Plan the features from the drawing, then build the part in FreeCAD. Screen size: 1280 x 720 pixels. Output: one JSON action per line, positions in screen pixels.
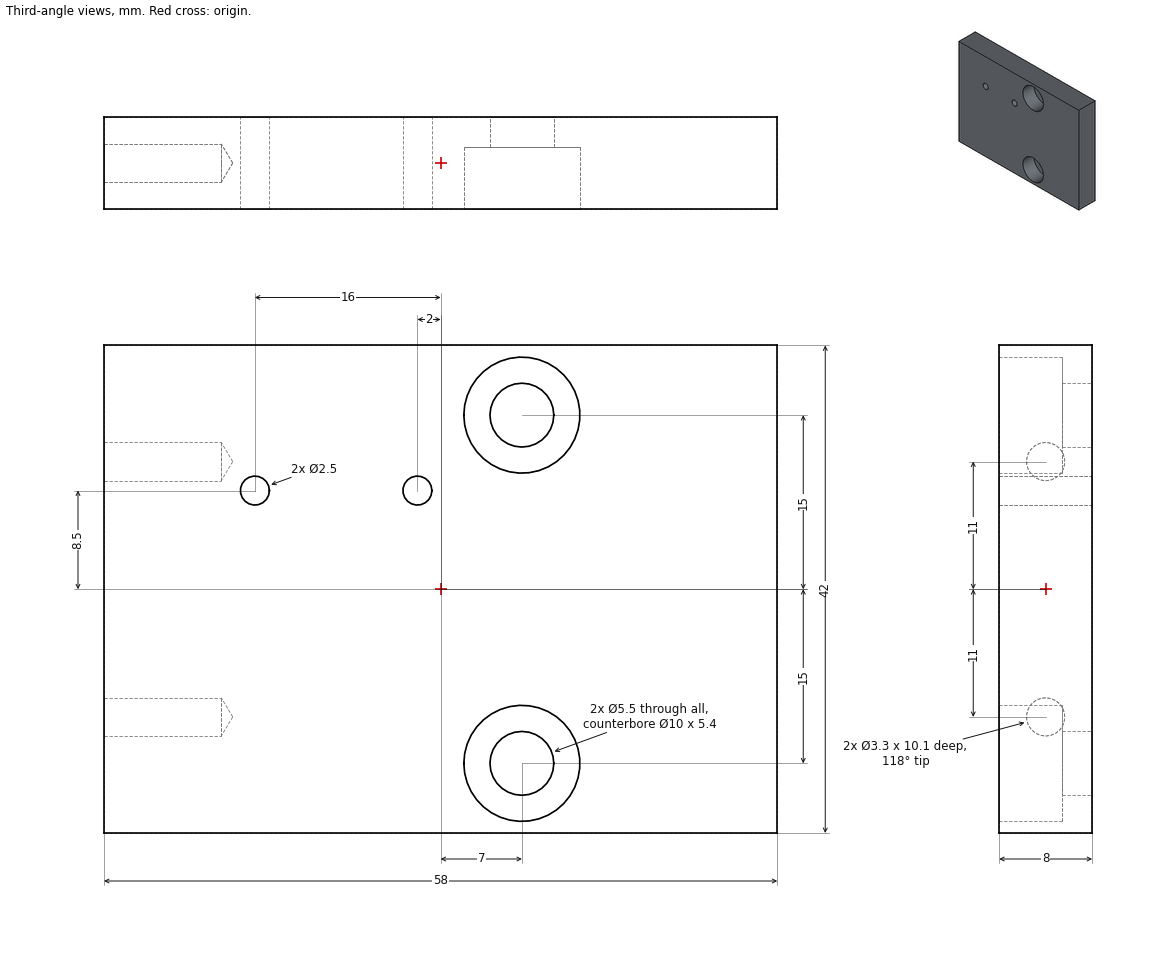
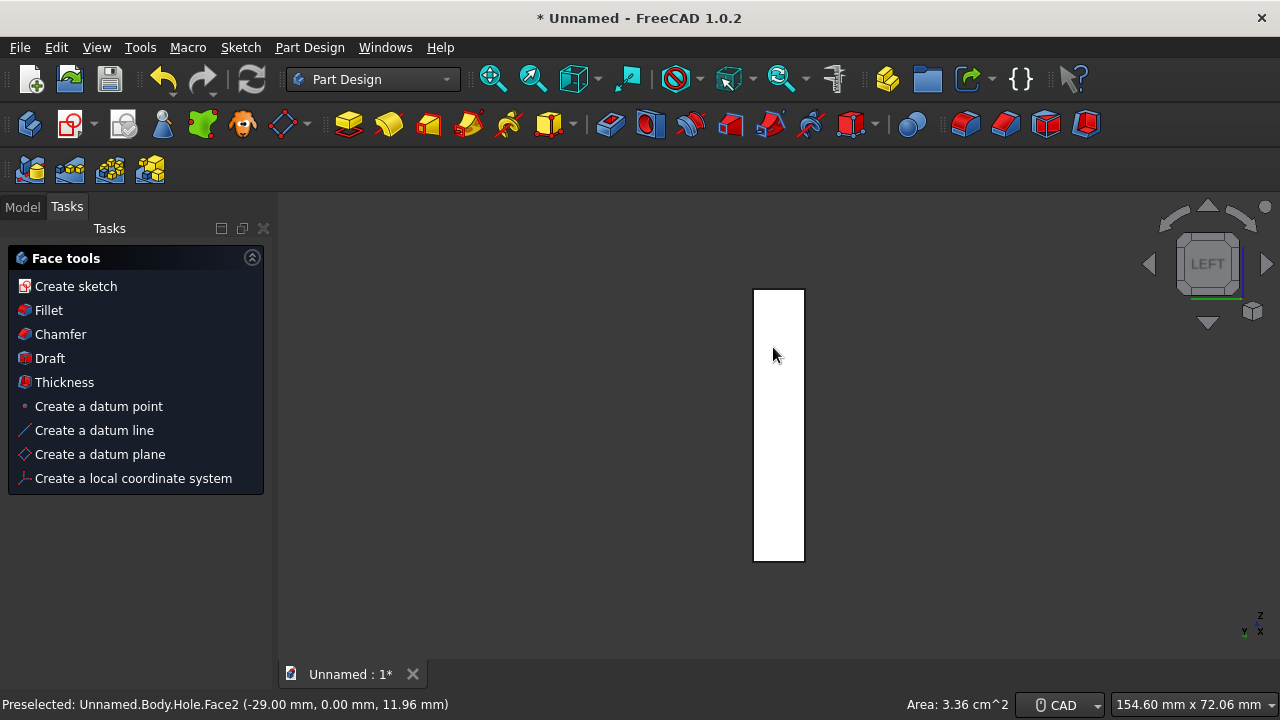
{"action": "left_click", "coordinate": [70, 124]}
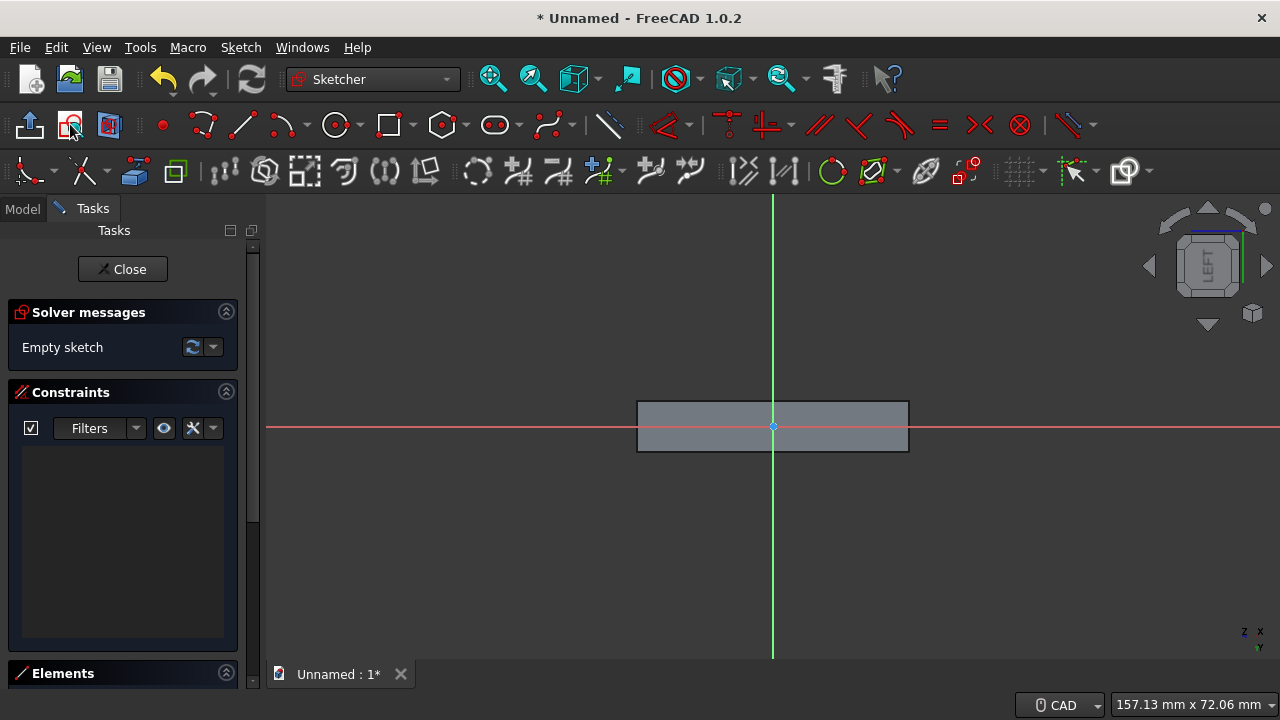
{"action": "scroll", "coordinate": [803, 427], "scroll_direction": "up", "scroll_amount": 6}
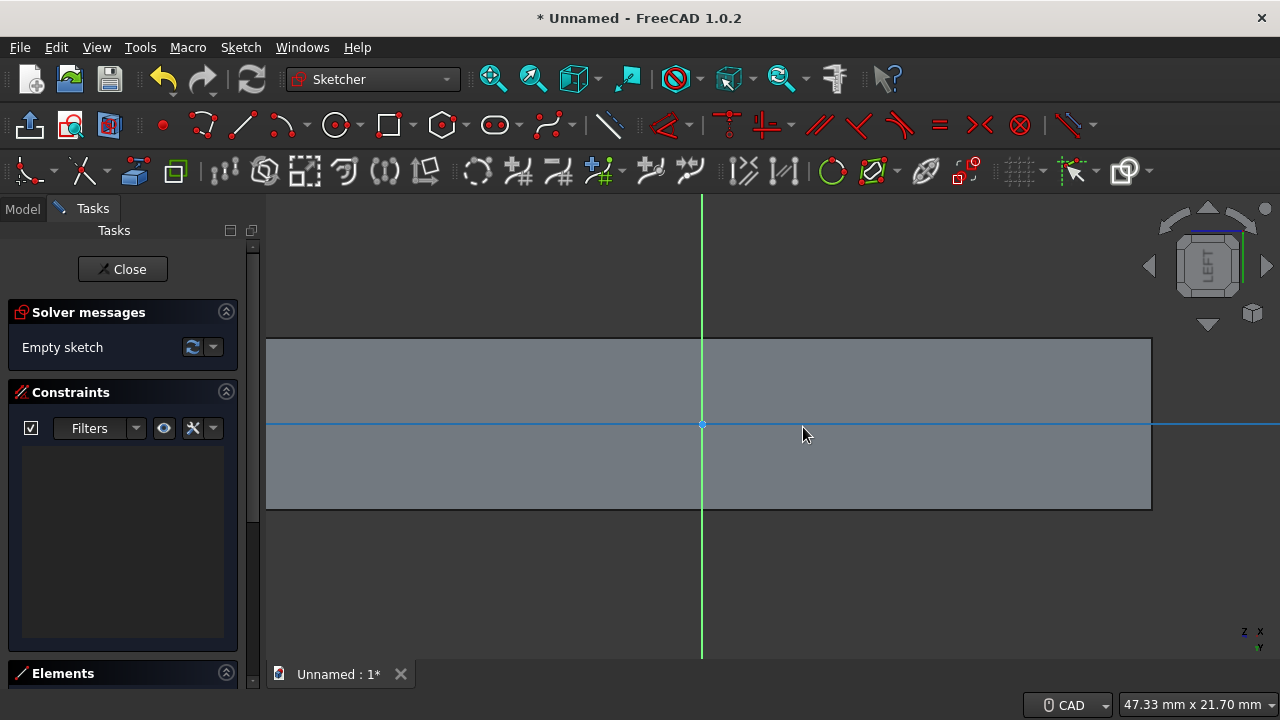
{"action": "left_click", "coordinate": [336, 126]}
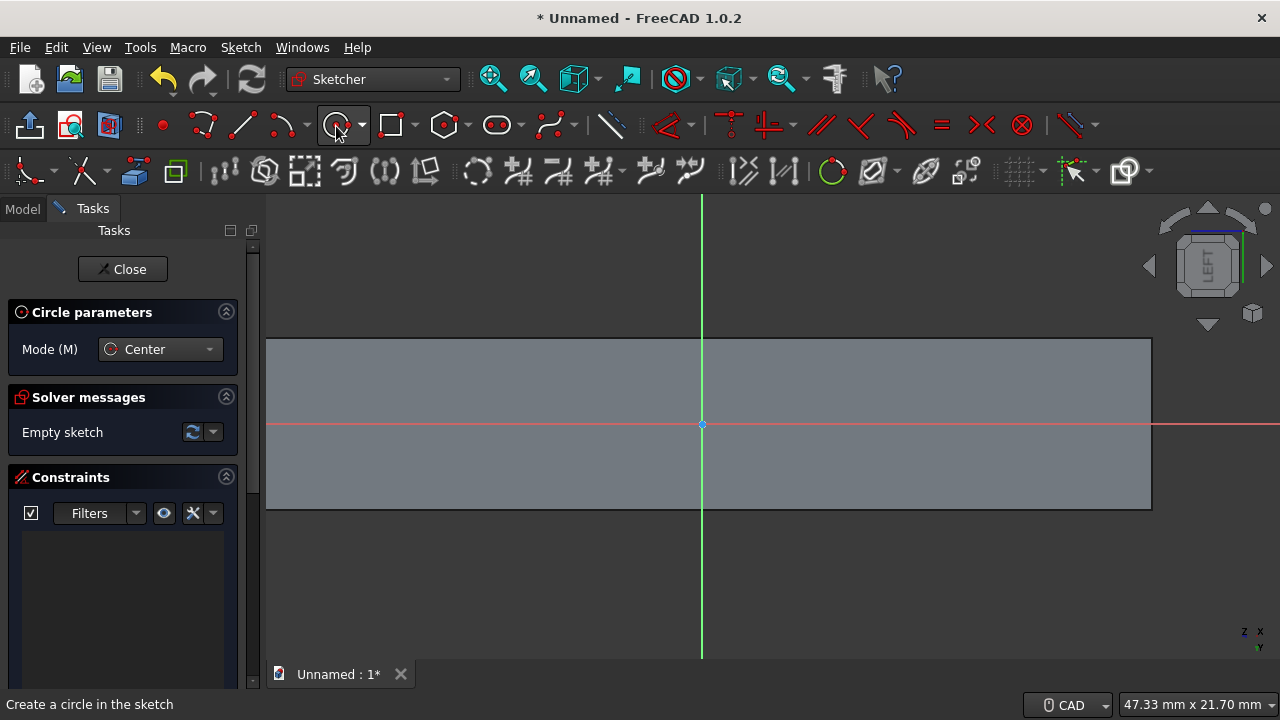
{"action": "left_click", "coordinate": [938, 424]}
{"action": "left_click", "coordinate": [963, 399]}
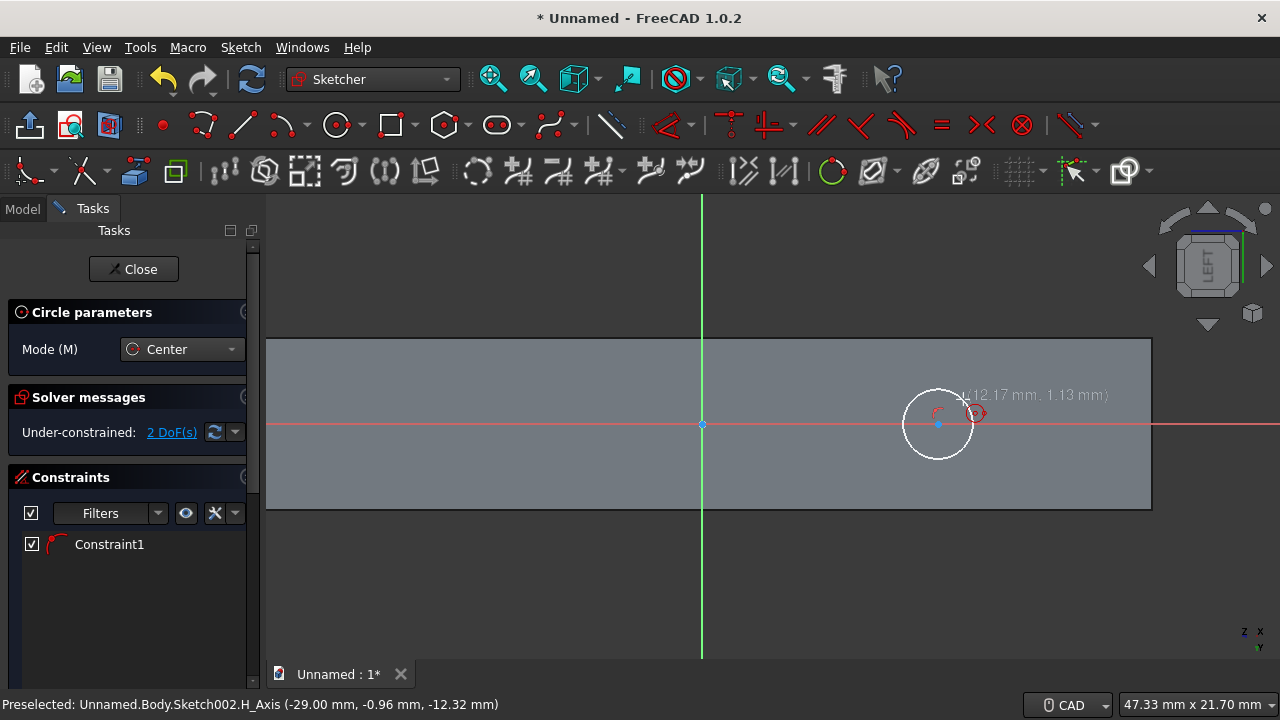
{"action": "left_click", "coordinate": [466, 424]}
{"action": "left_click", "coordinate": [491, 399]}
{"action": "key", "text": "Escape"}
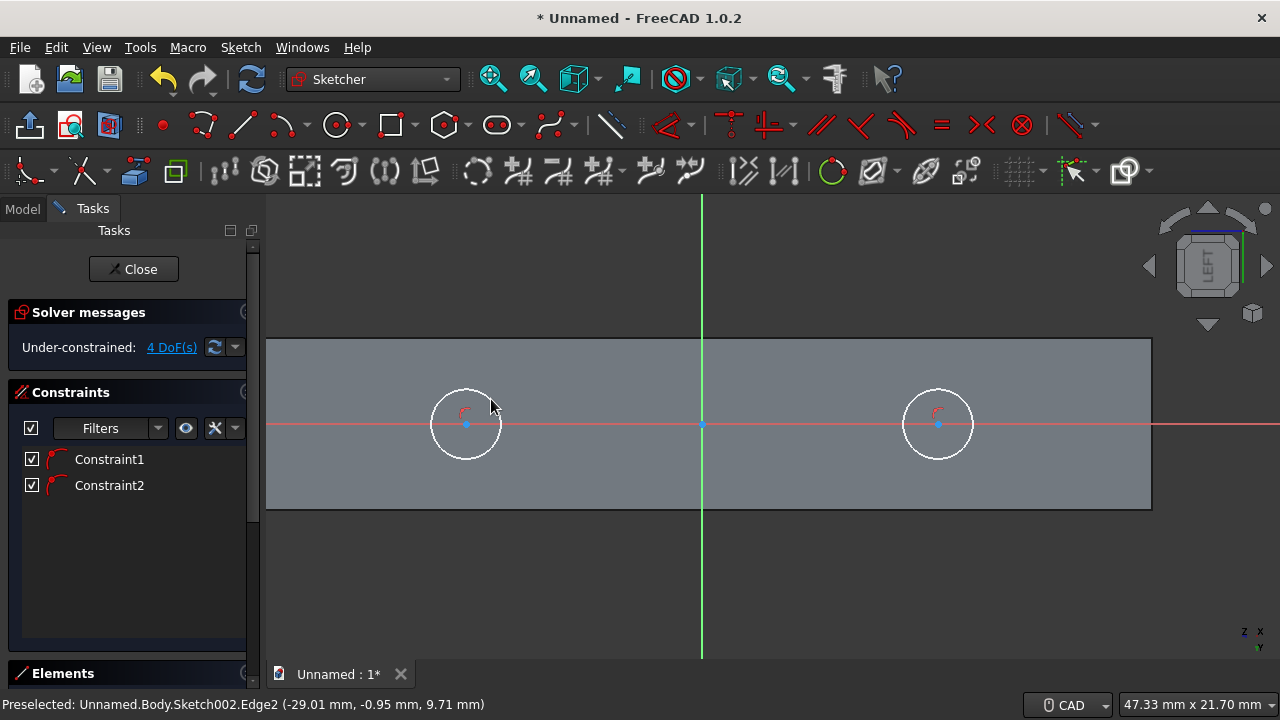
{"action": "left_click", "coordinate": [963, 400]}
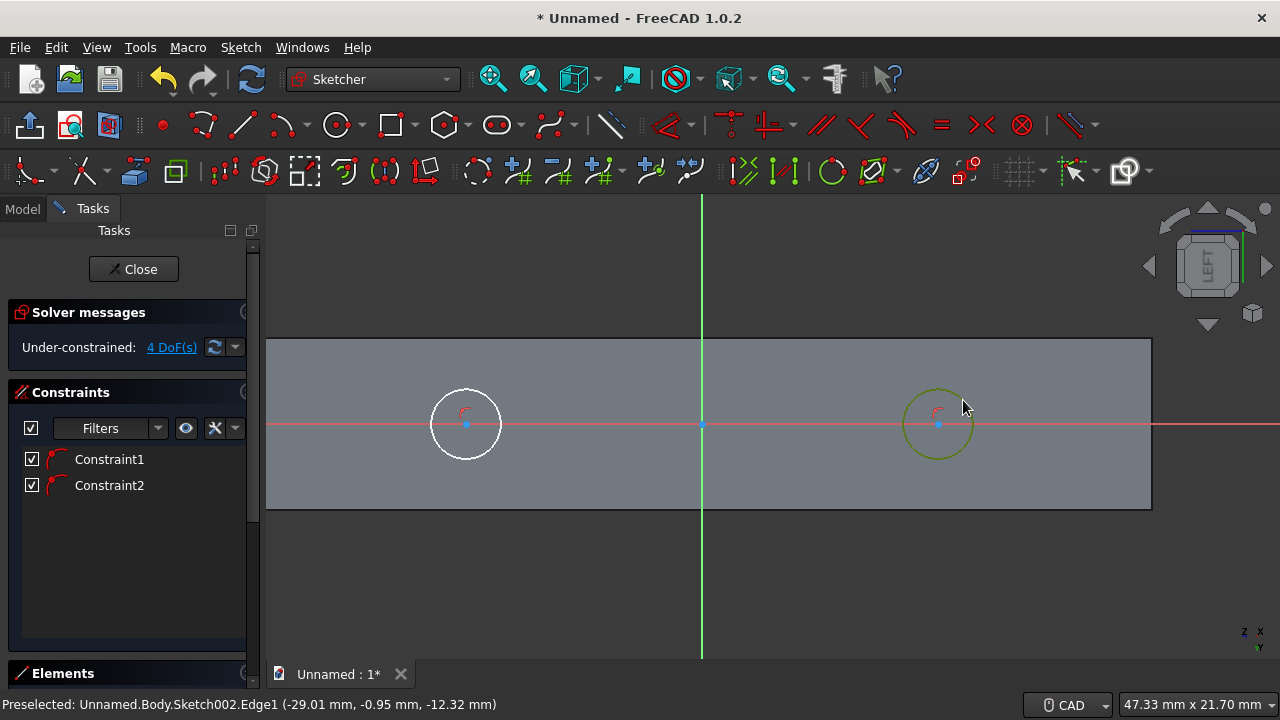
{"action": "left_click", "coordinate": [491, 400]}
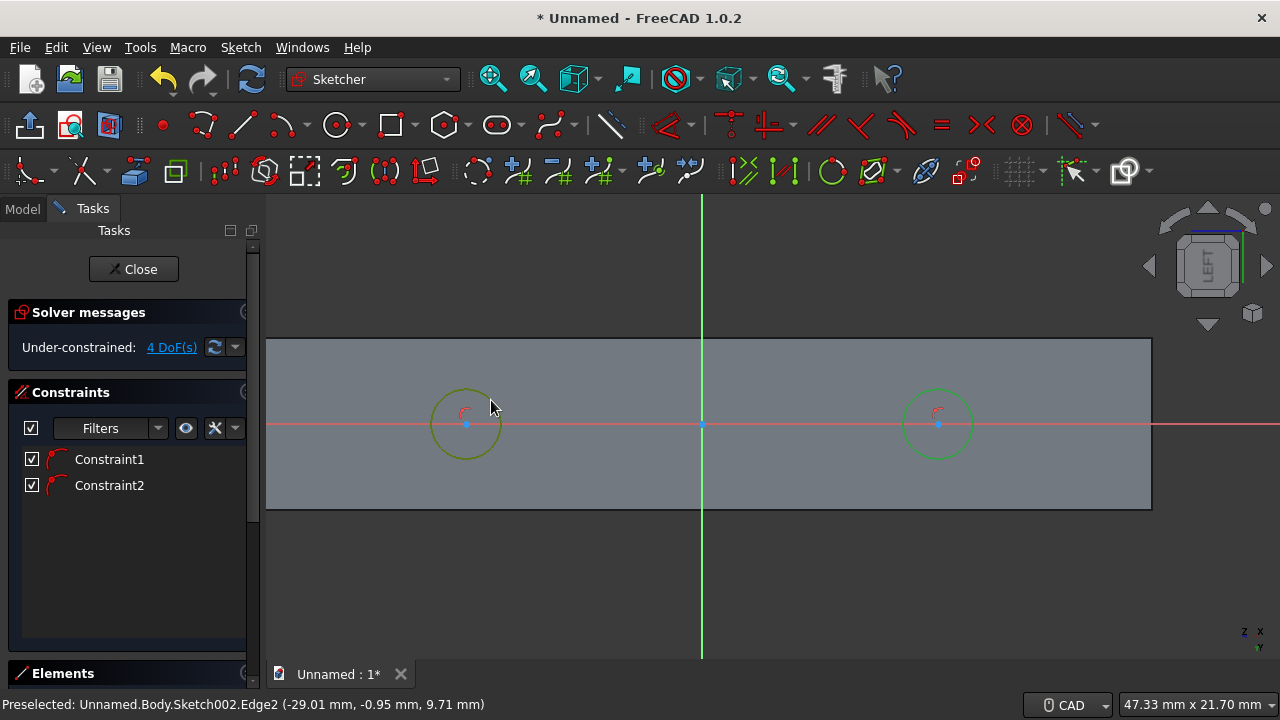
{"action": "left_click", "coordinate": [942, 126]}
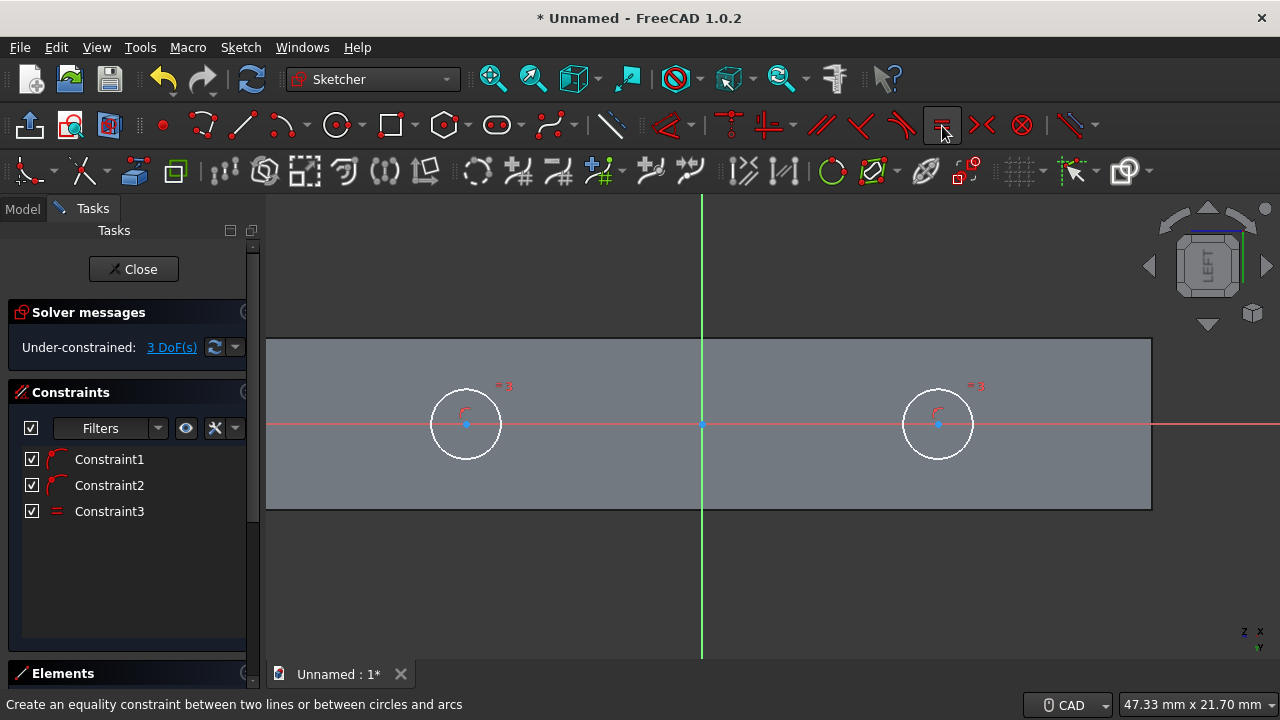
{"action": "left_click", "coordinate": [666, 126]}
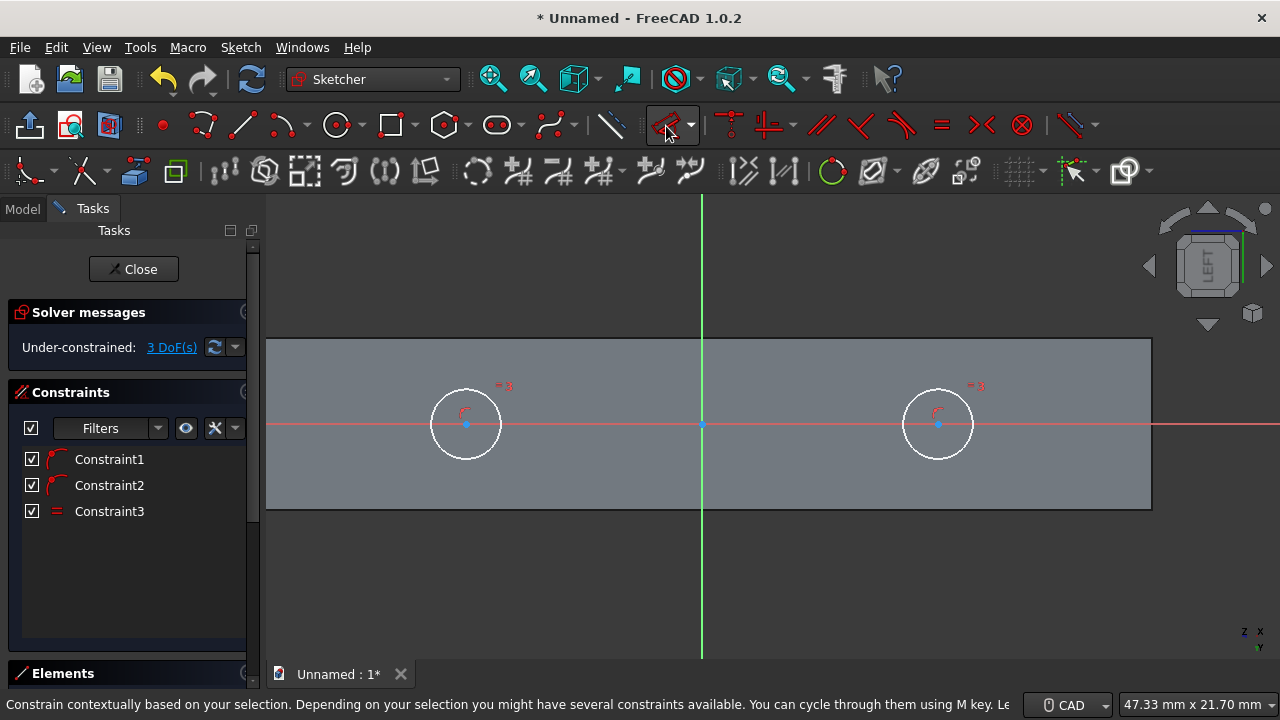
{"action": "left_click", "coordinate": [963, 400]}
{"action": "left_click", "coordinate": [986, 378]}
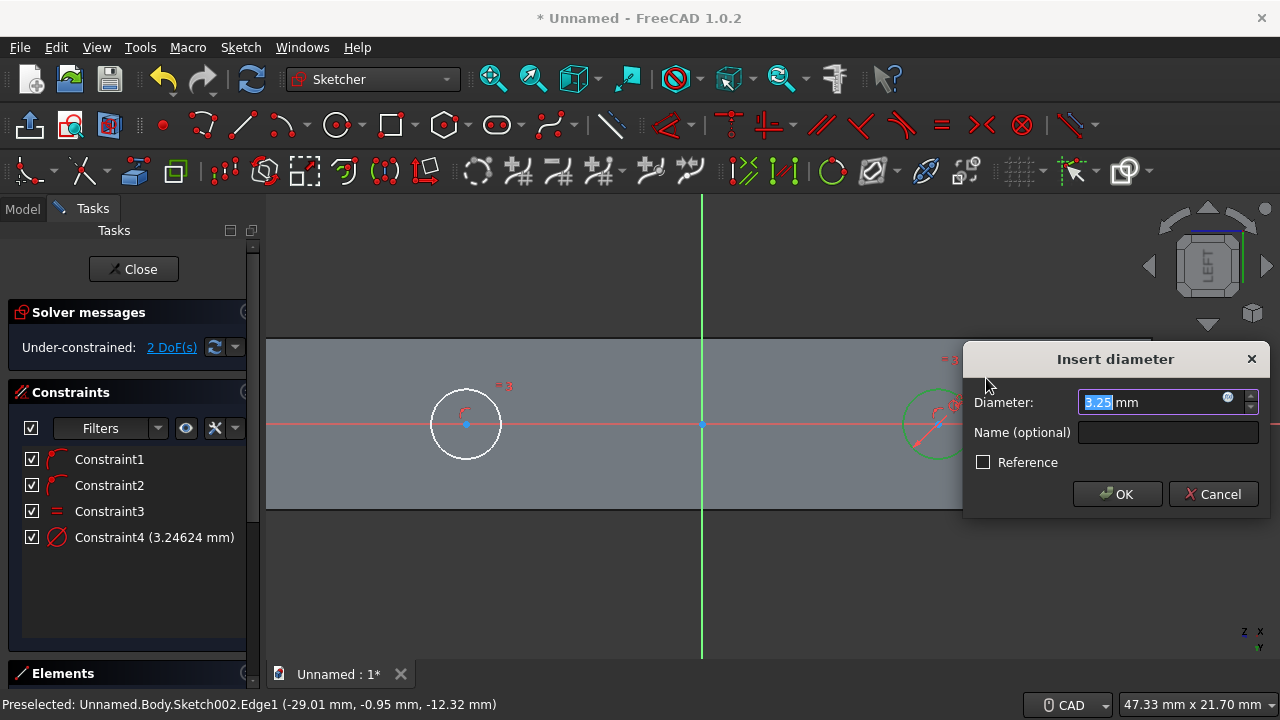
{"action": "type", "text": "3.3"}
{"action": "key", "text": "Return"}